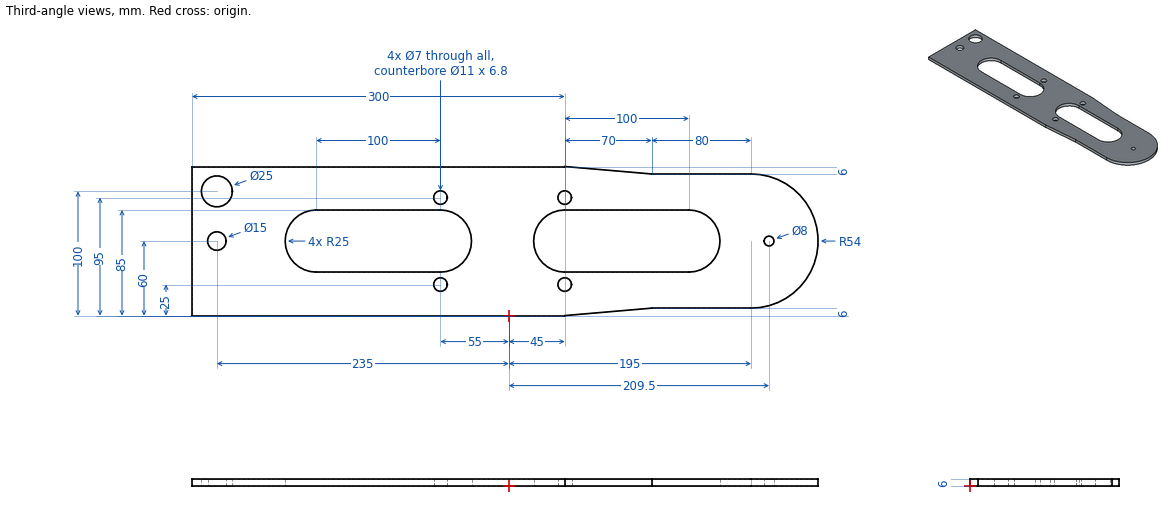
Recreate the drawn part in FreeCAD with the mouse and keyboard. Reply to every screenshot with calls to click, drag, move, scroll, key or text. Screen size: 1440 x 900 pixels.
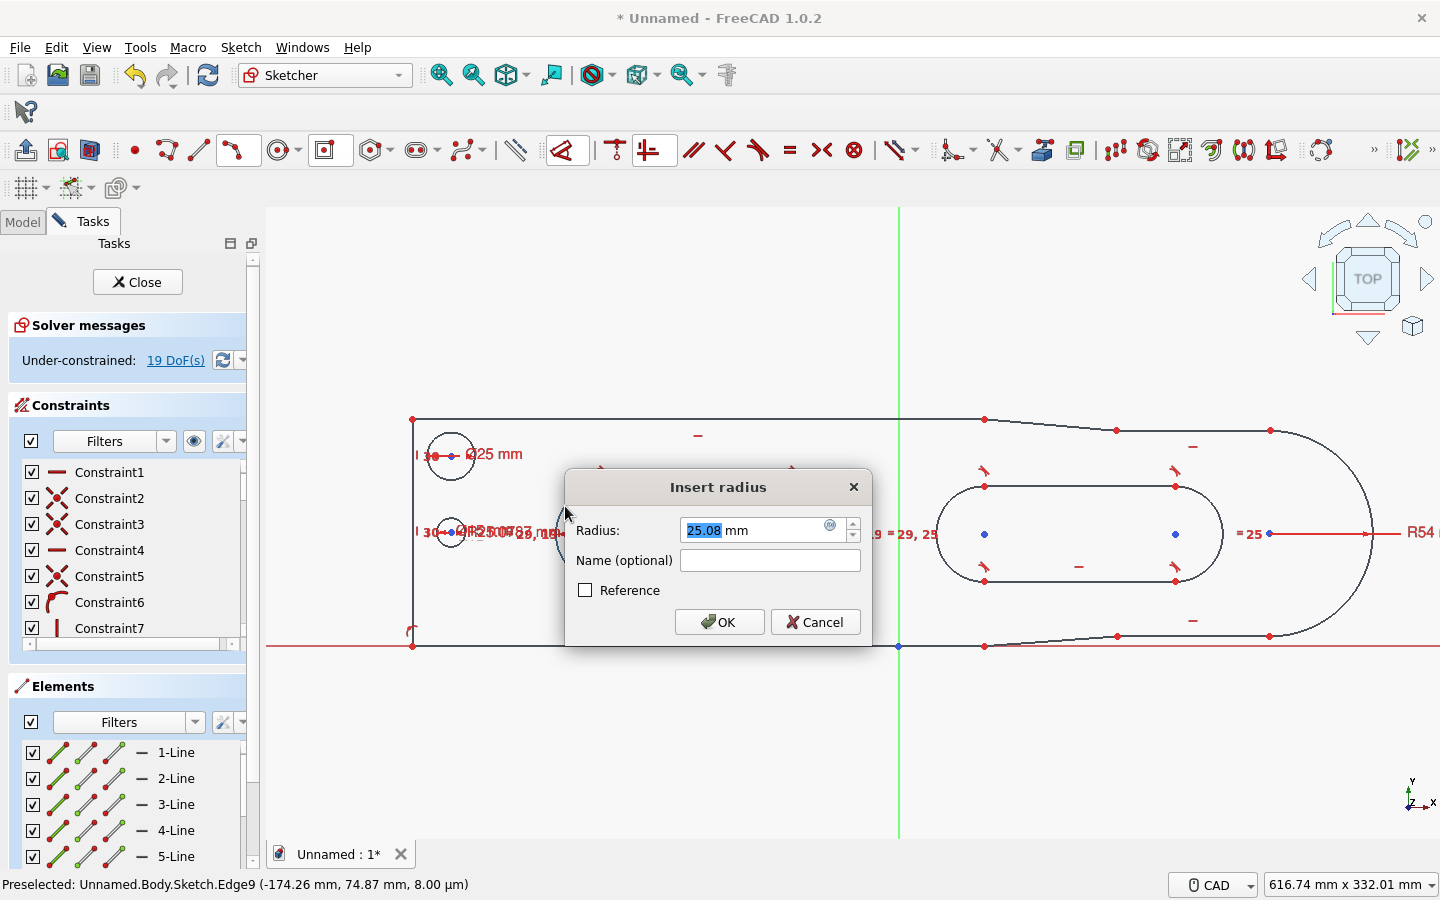
text(25)
key(Return)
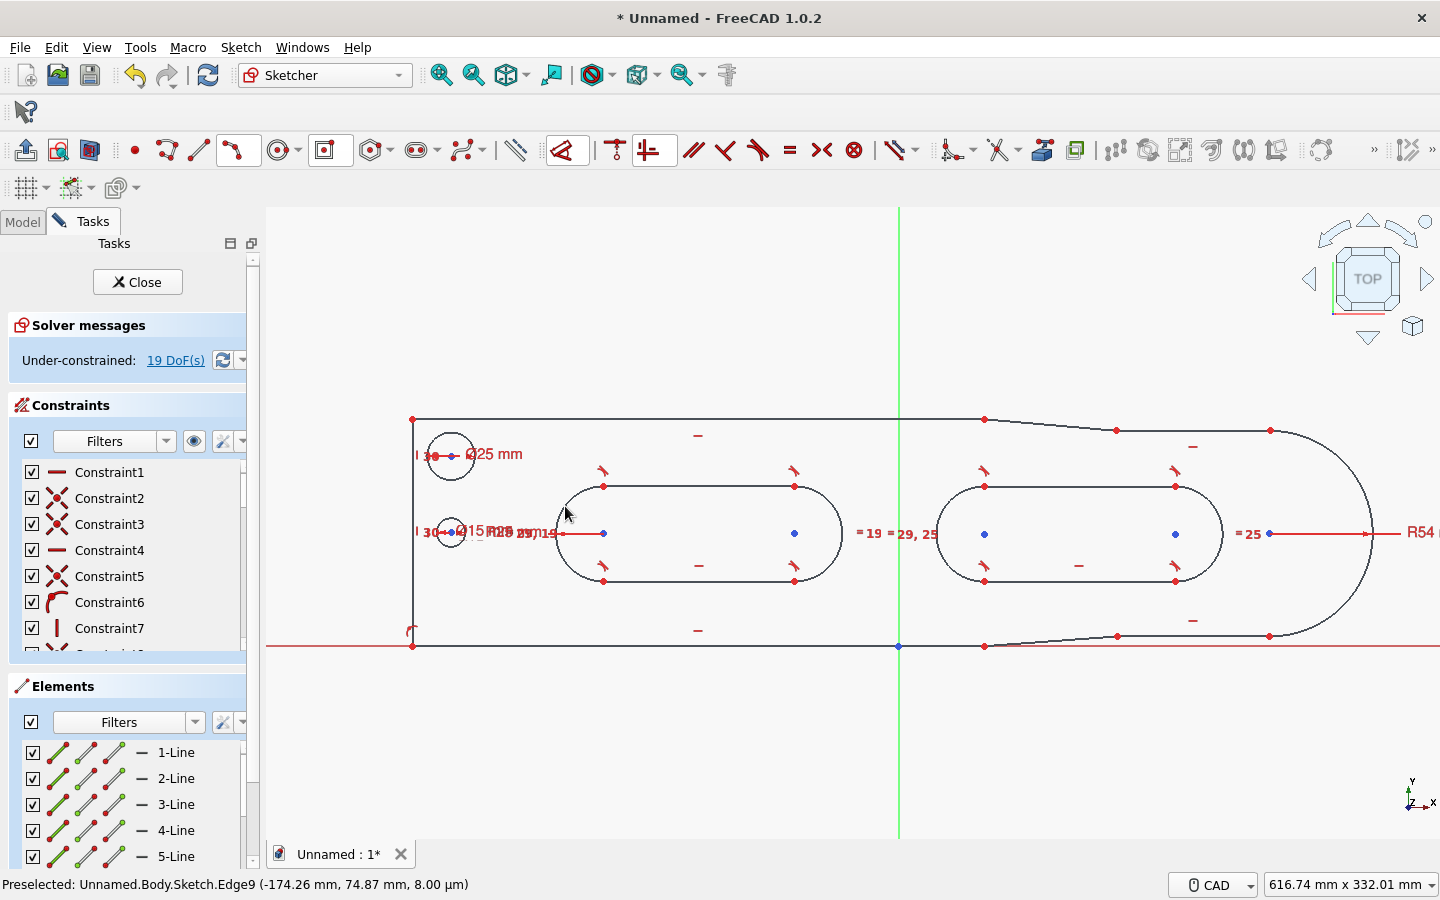
click(1224, 431)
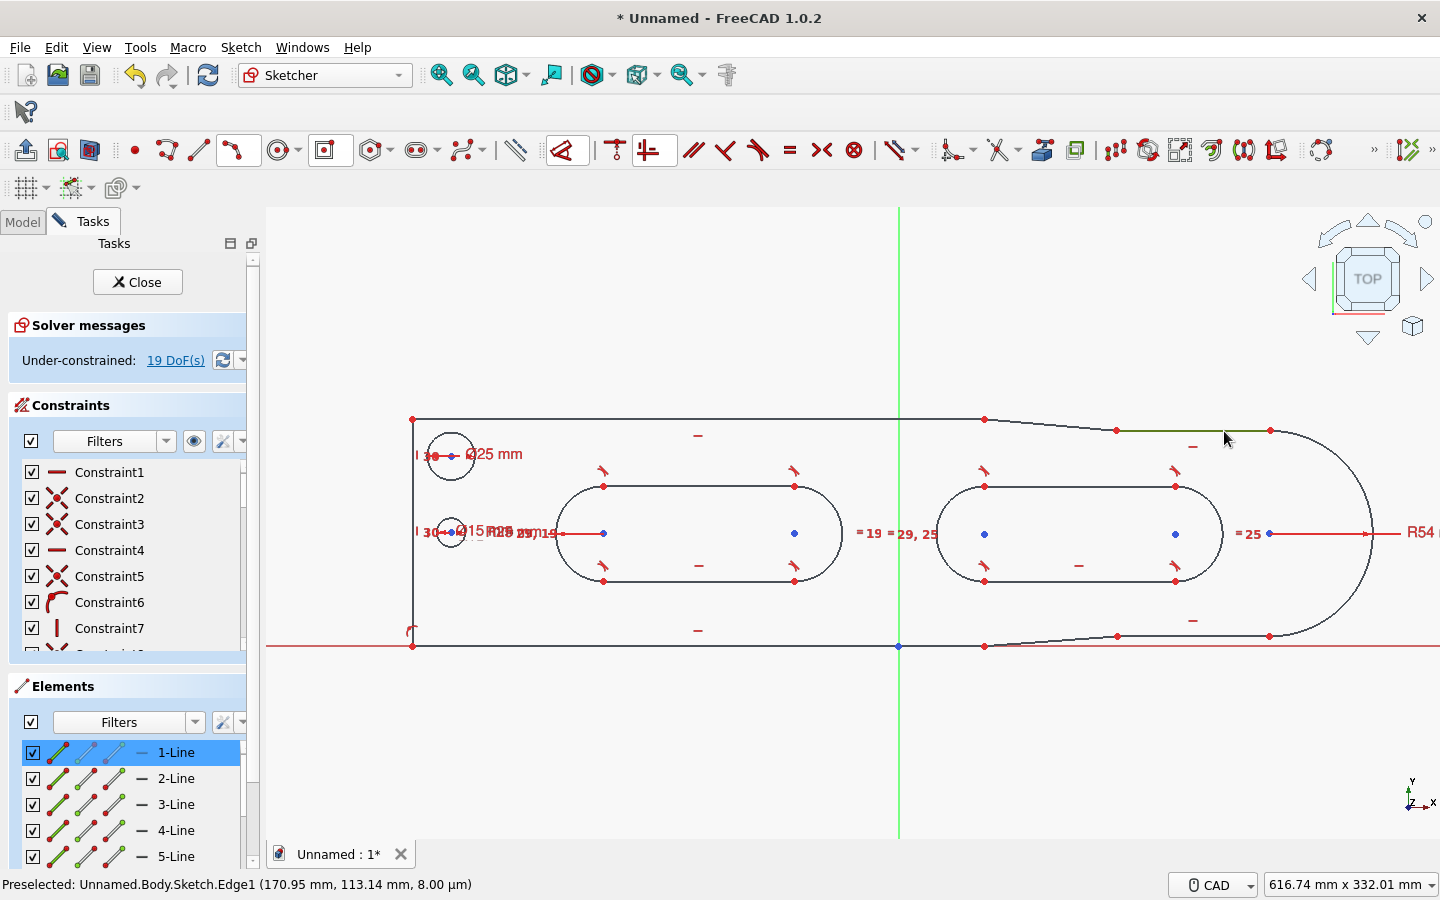
key(l)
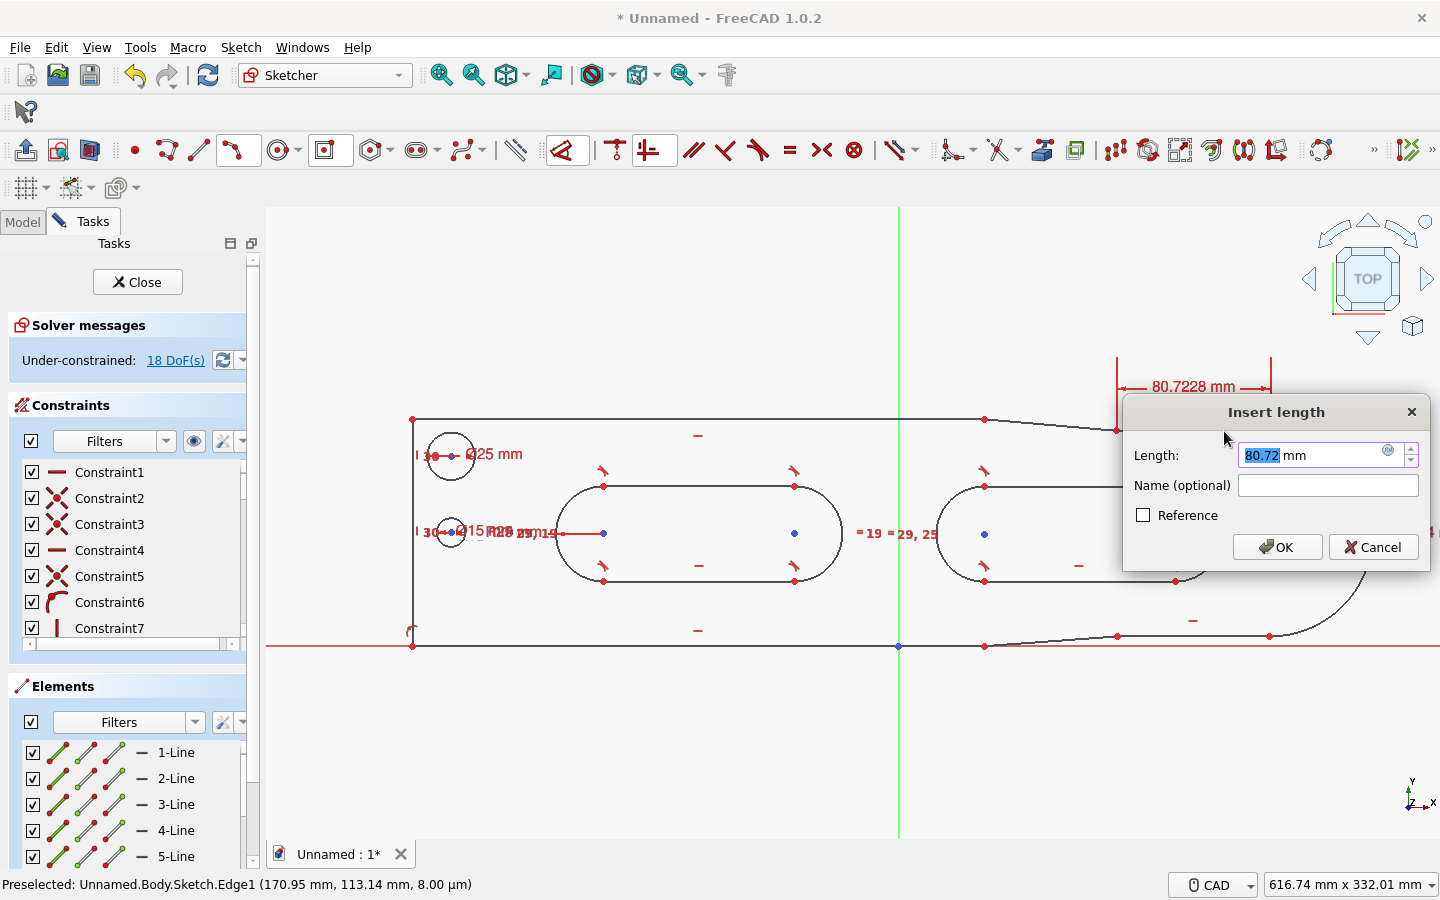
text(80)
key(Return)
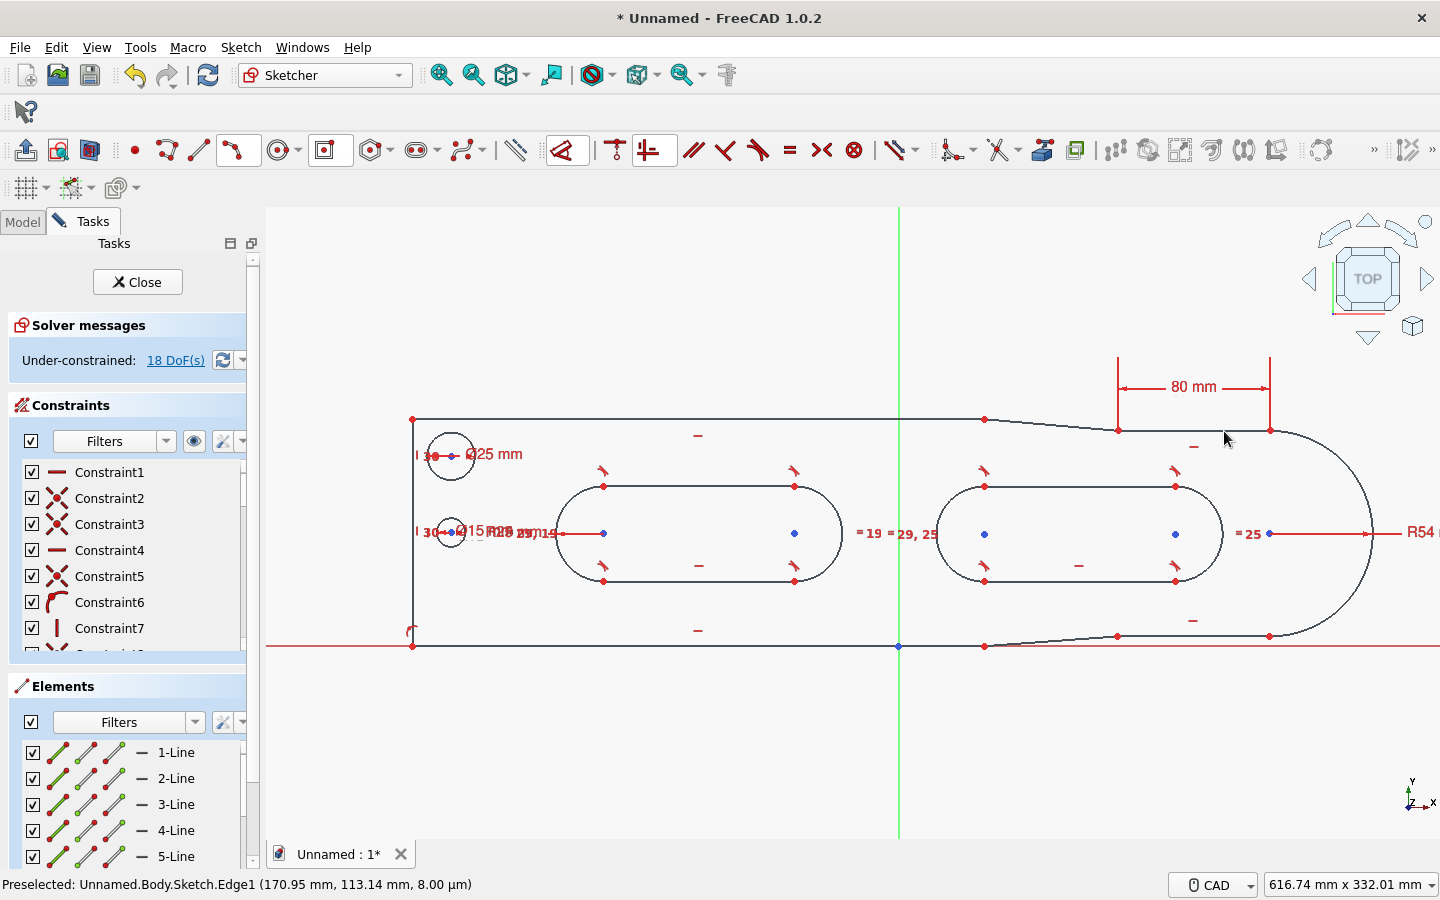
scroll(1163, 636, up, 2)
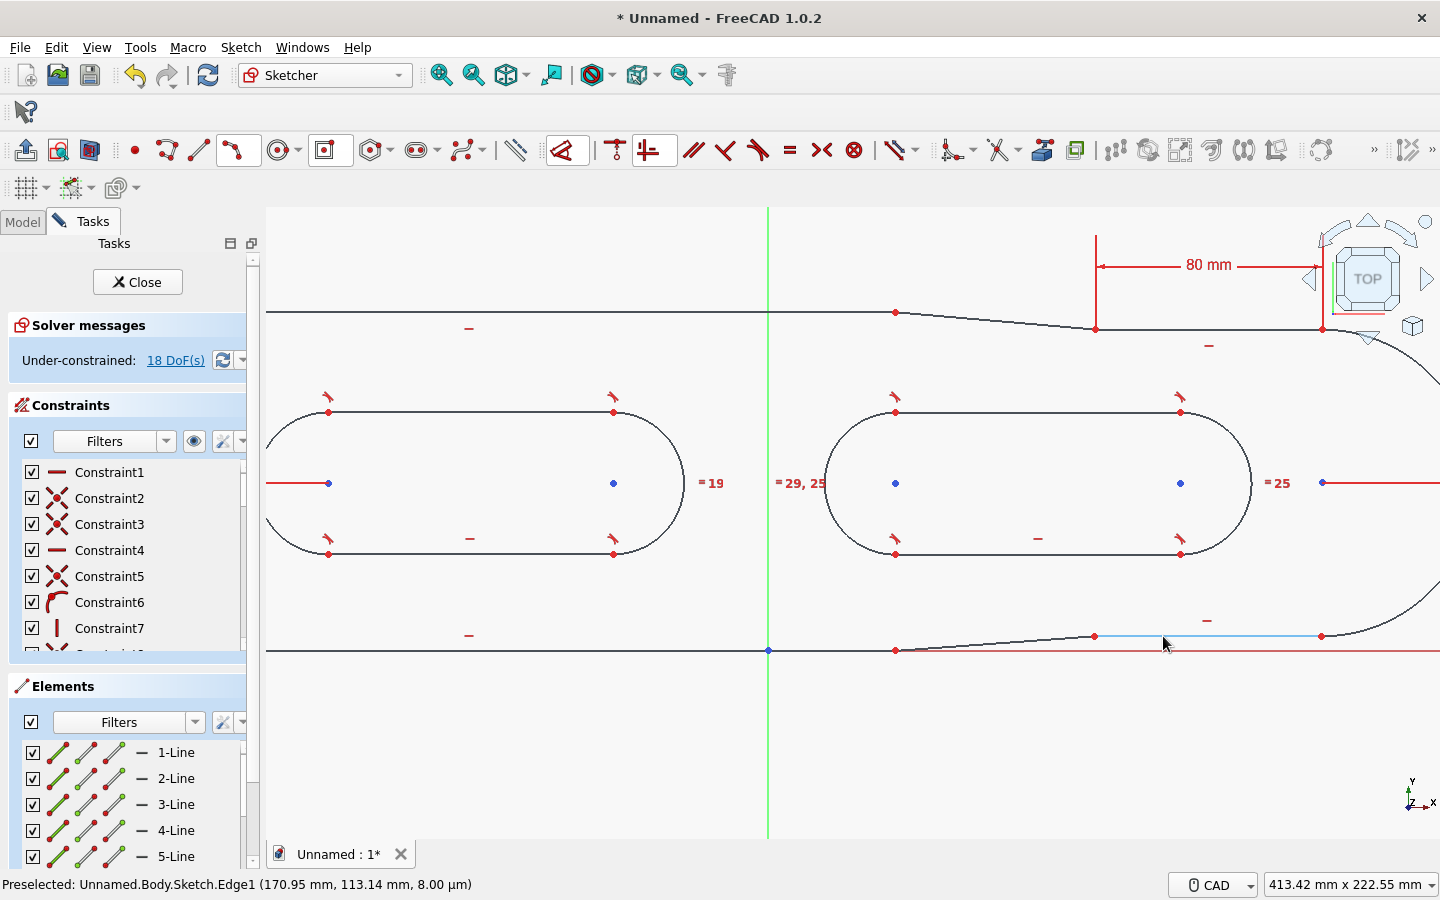
click(1163, 636)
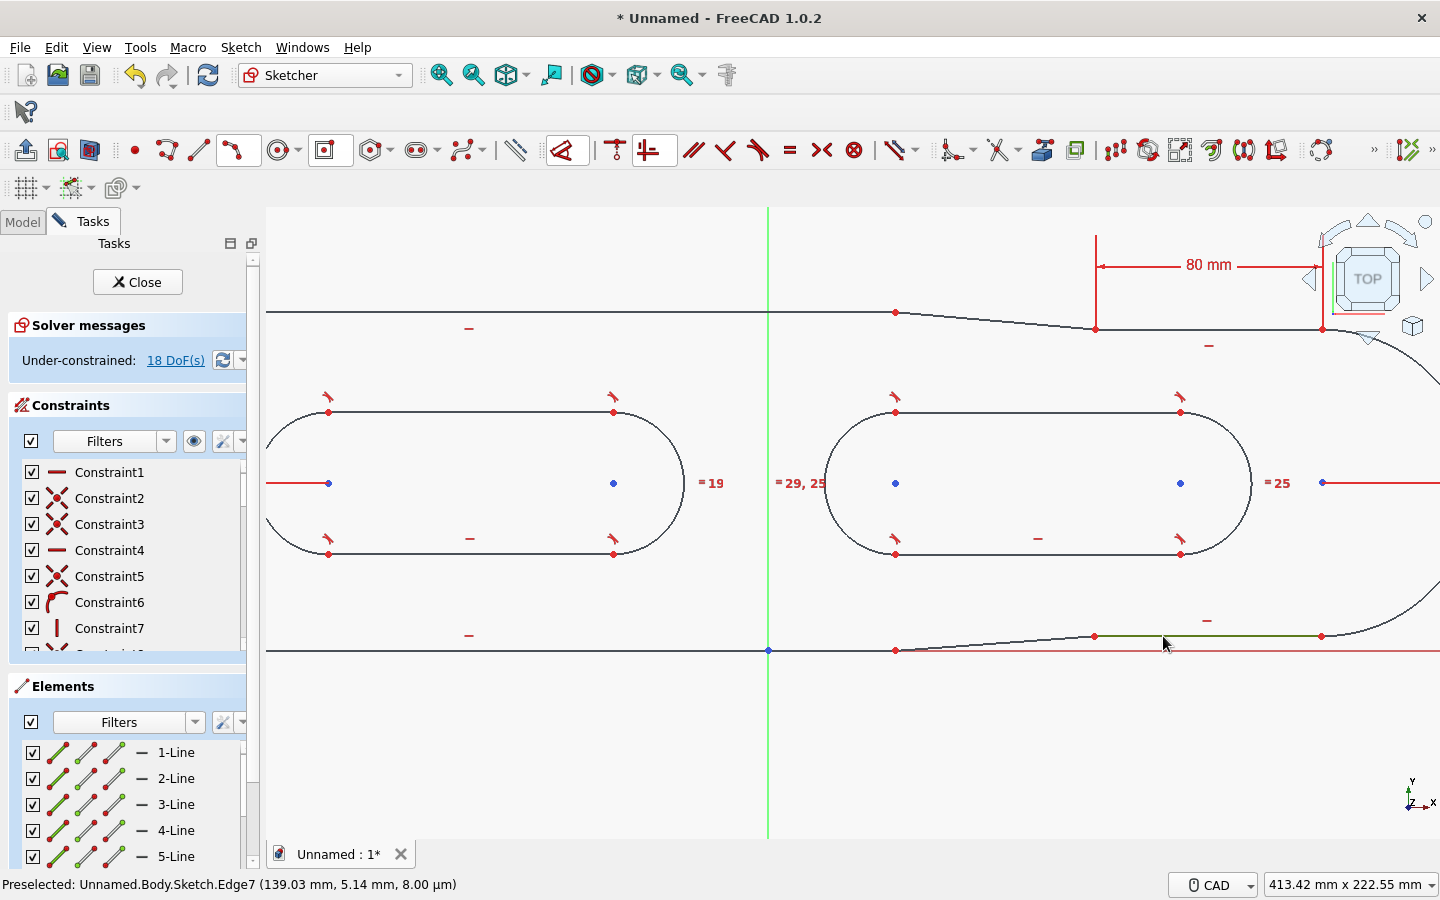
key(l)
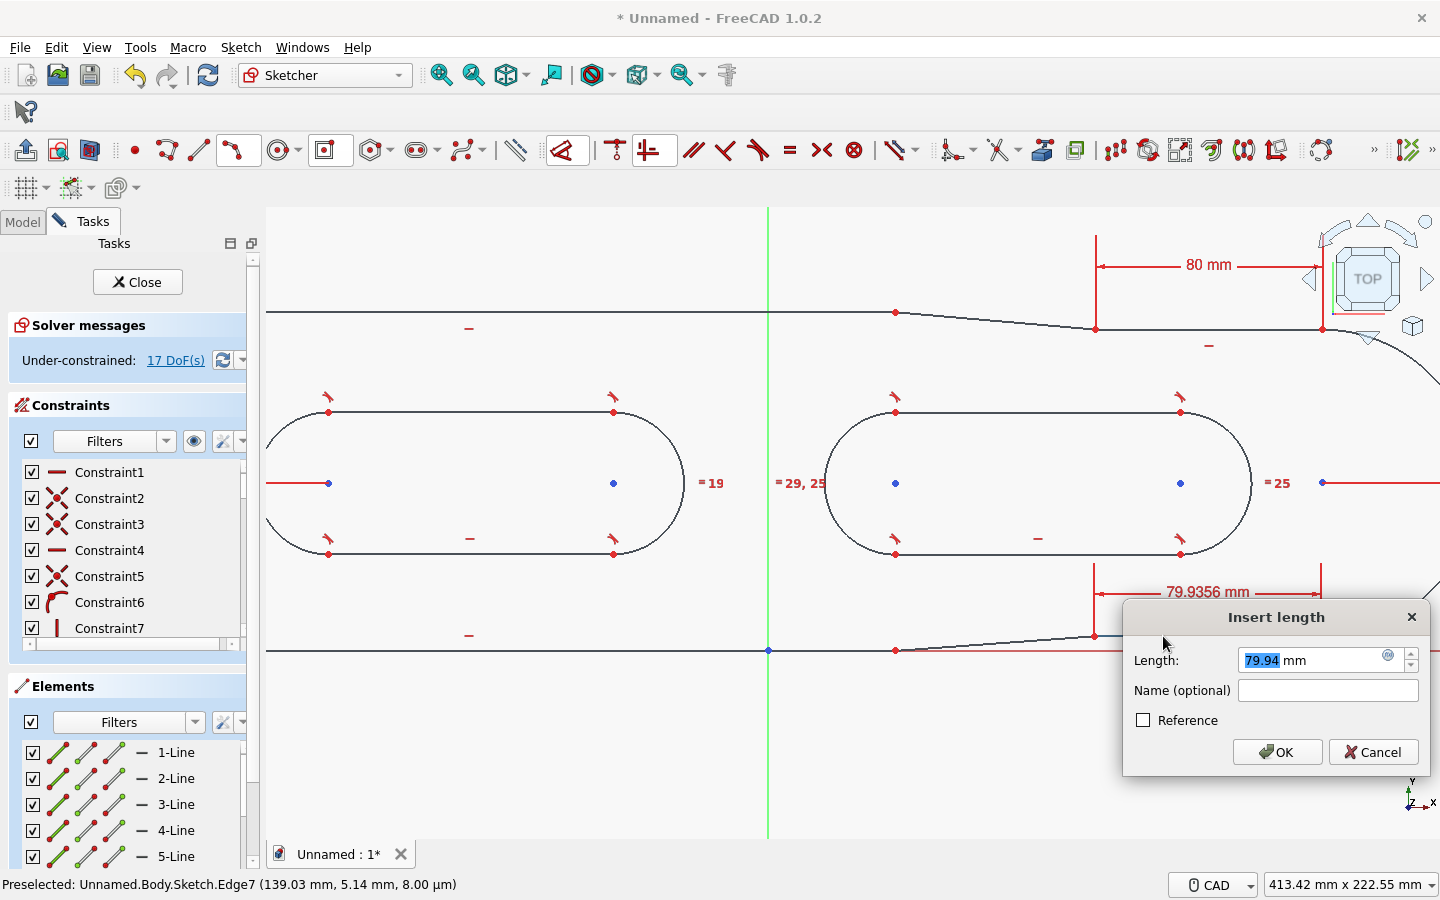
text(80)
key(Return)